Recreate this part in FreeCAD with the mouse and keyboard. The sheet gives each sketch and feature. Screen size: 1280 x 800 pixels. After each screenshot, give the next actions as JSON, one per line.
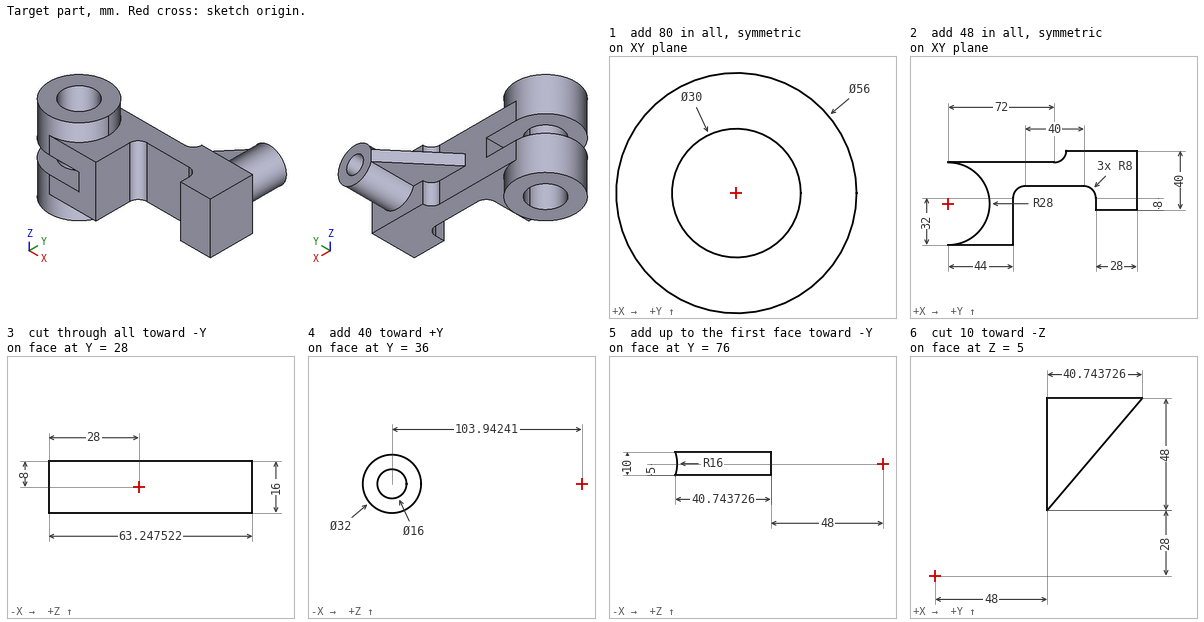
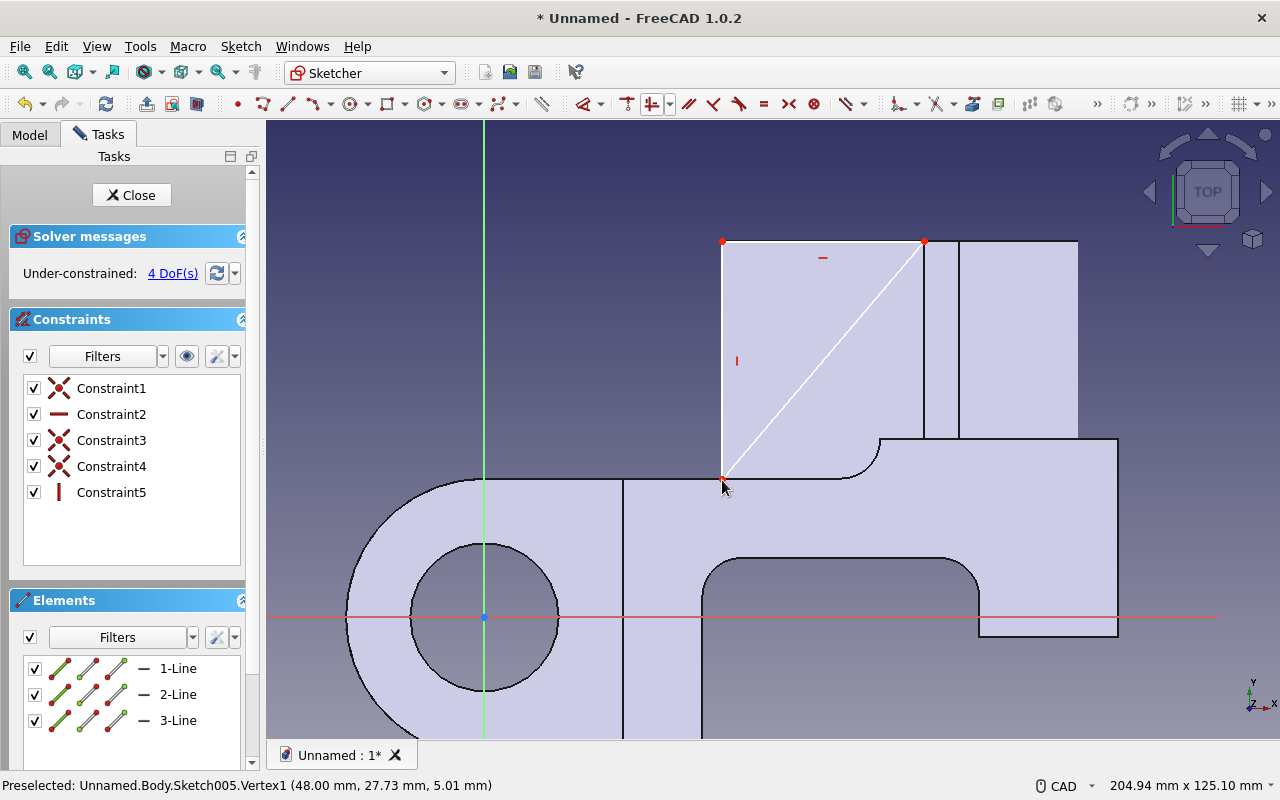
{"action": "left_click", "coordinate": [582, 104]}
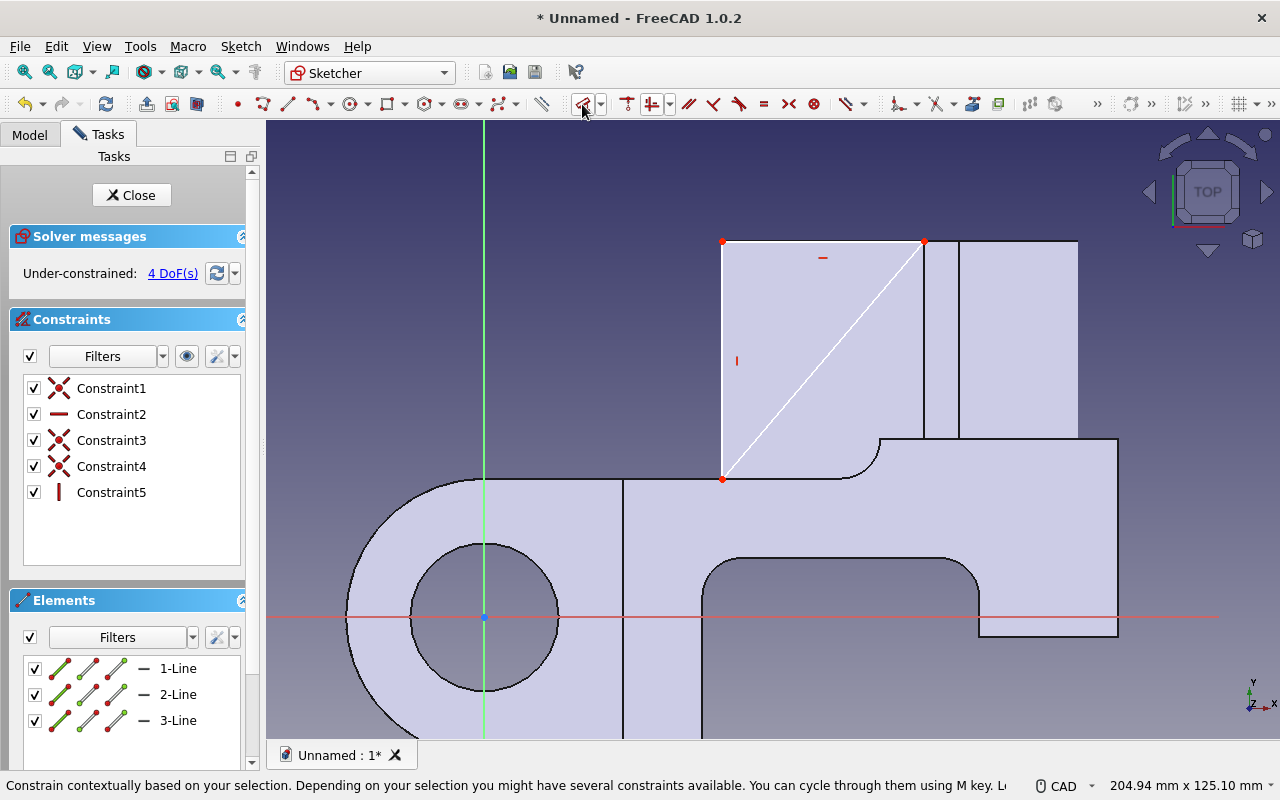
{"action": "left_click", "coordinate": [722, 313]}
{"action": "left_click", "coordinate": [756, 361]}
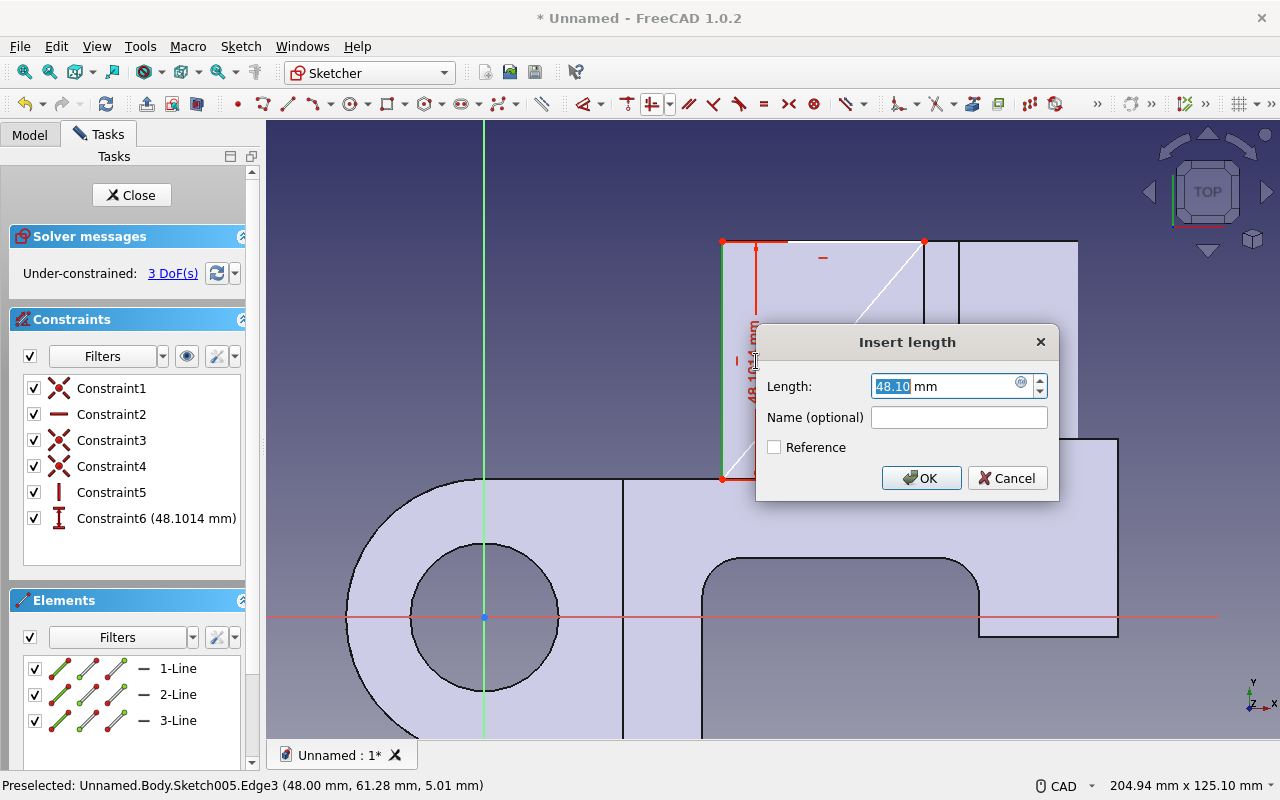
{"action": "type", "text": "48"}
{"action": "key", "text": "Return"}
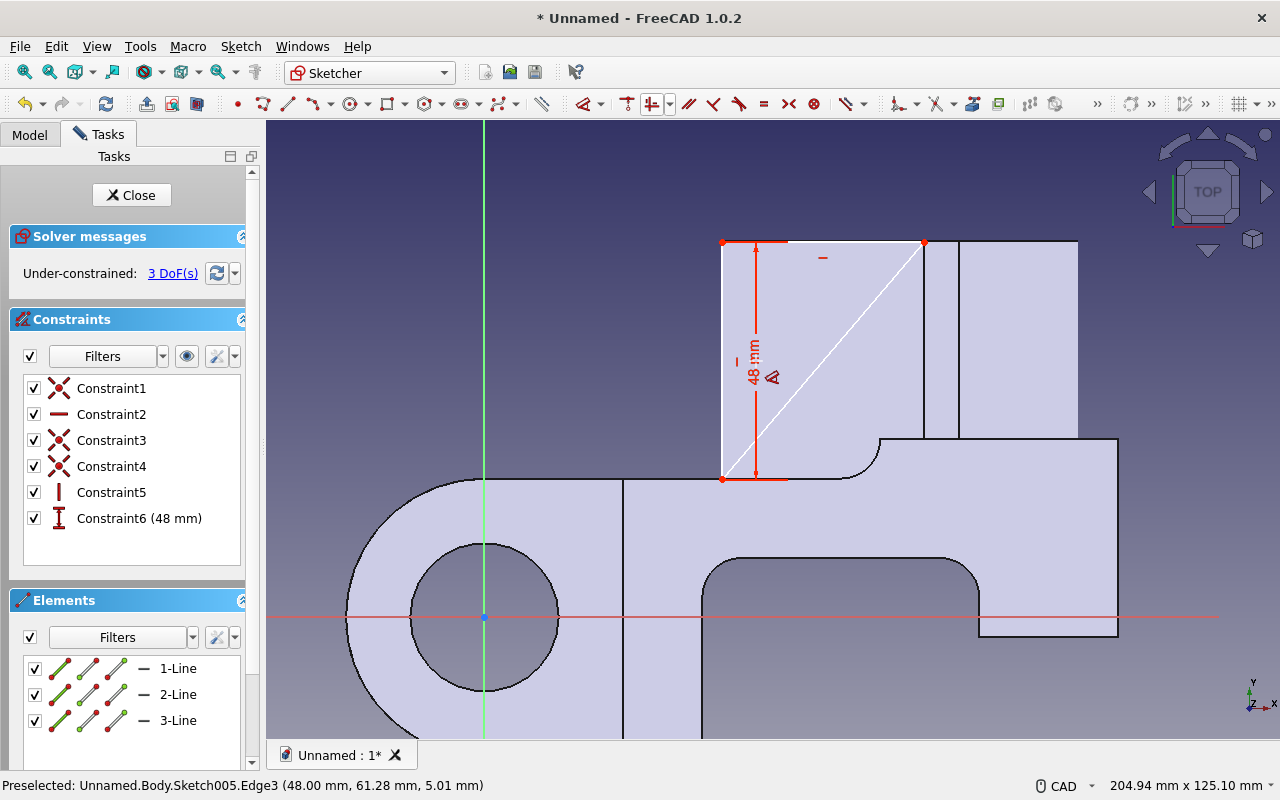
{"action": "left_click", "coordinate": [722, 480]}
{"action": "left_click", "coordinate": [603, 651]}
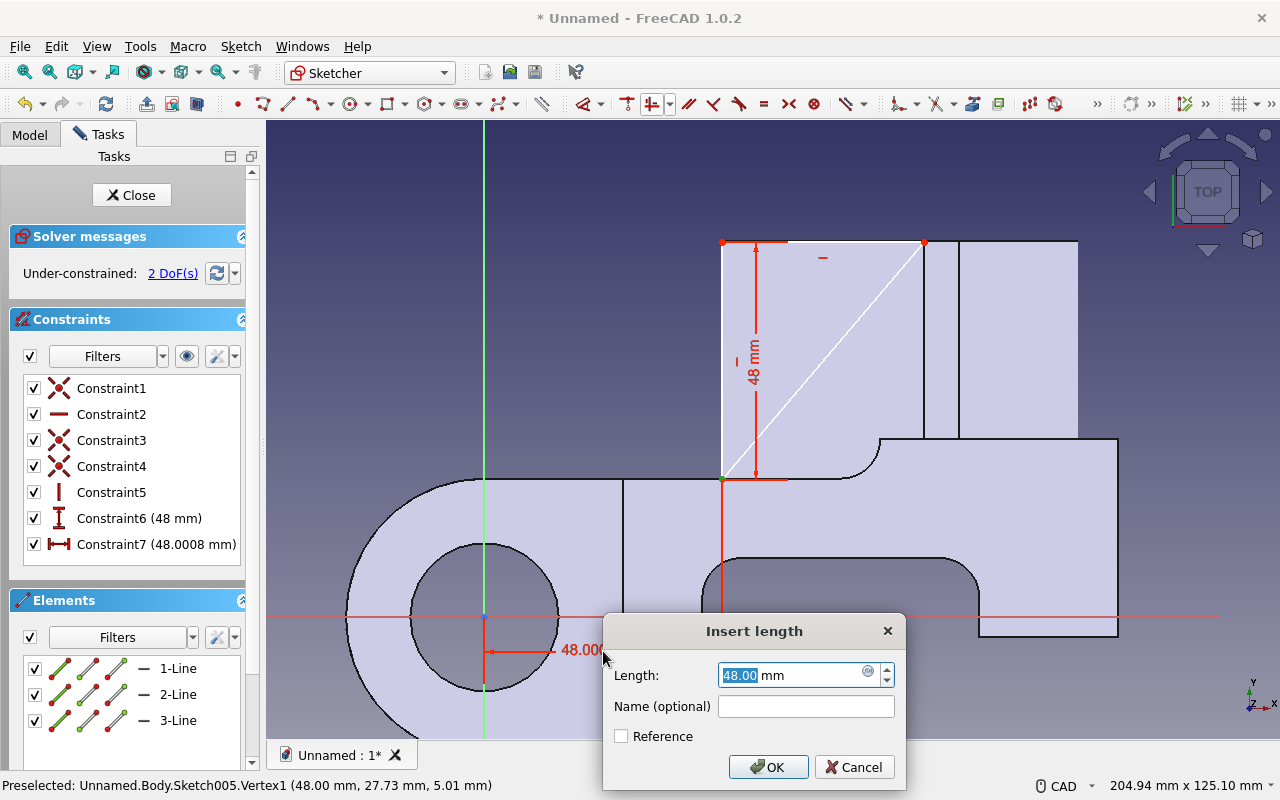
{"action": "type", "text": "48"}
{"action": "key", "text": "Return"}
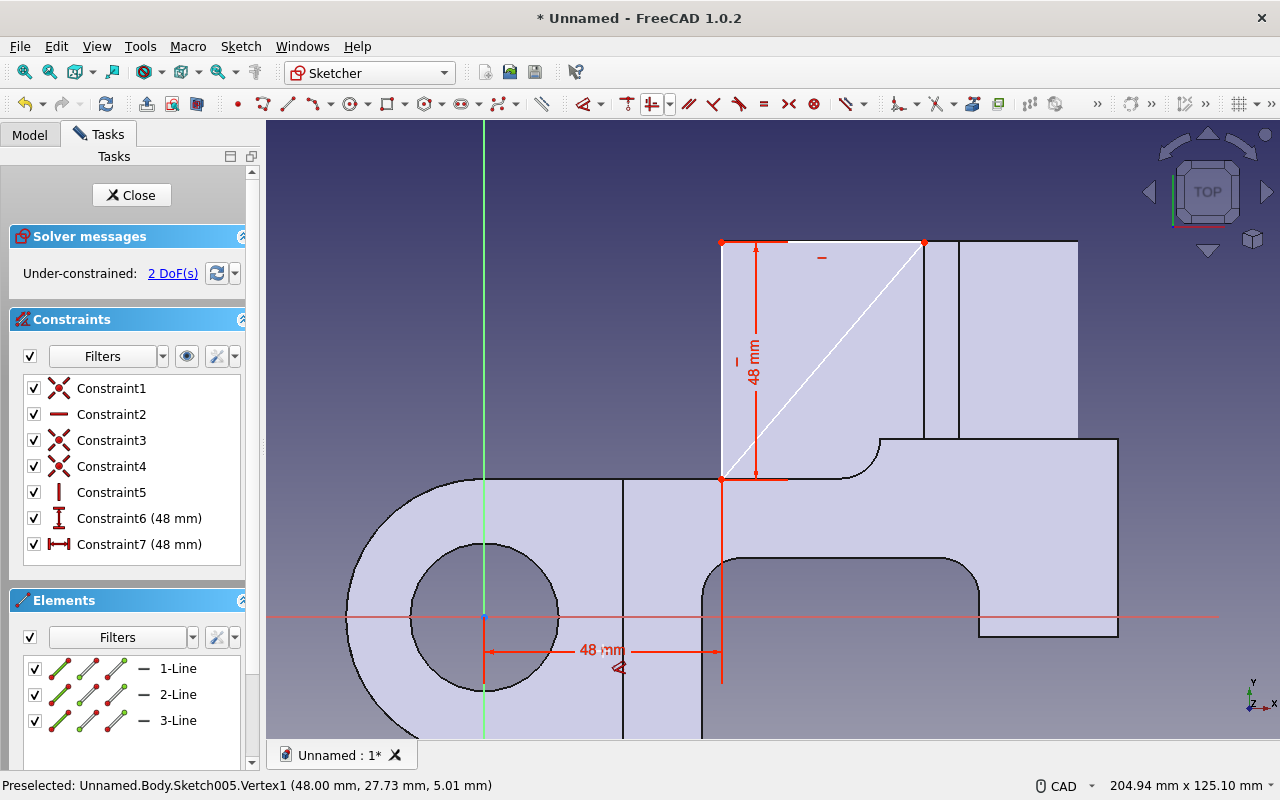
{"action": "left_click", "coordinate": [722, 480]}
{"action": "left_click", "coordinate": [450, 549]}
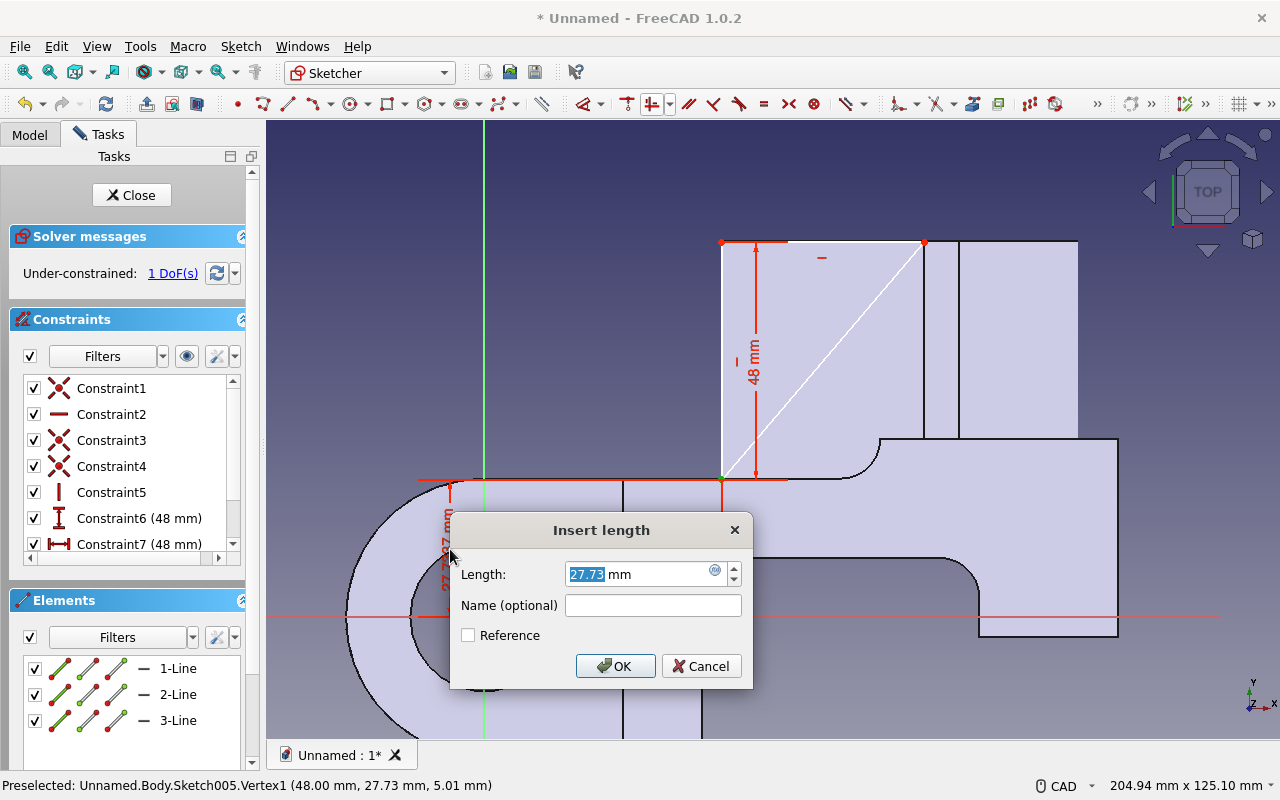
{"action": "type", "text": "28"}
{"action": "key", "text": "Return"}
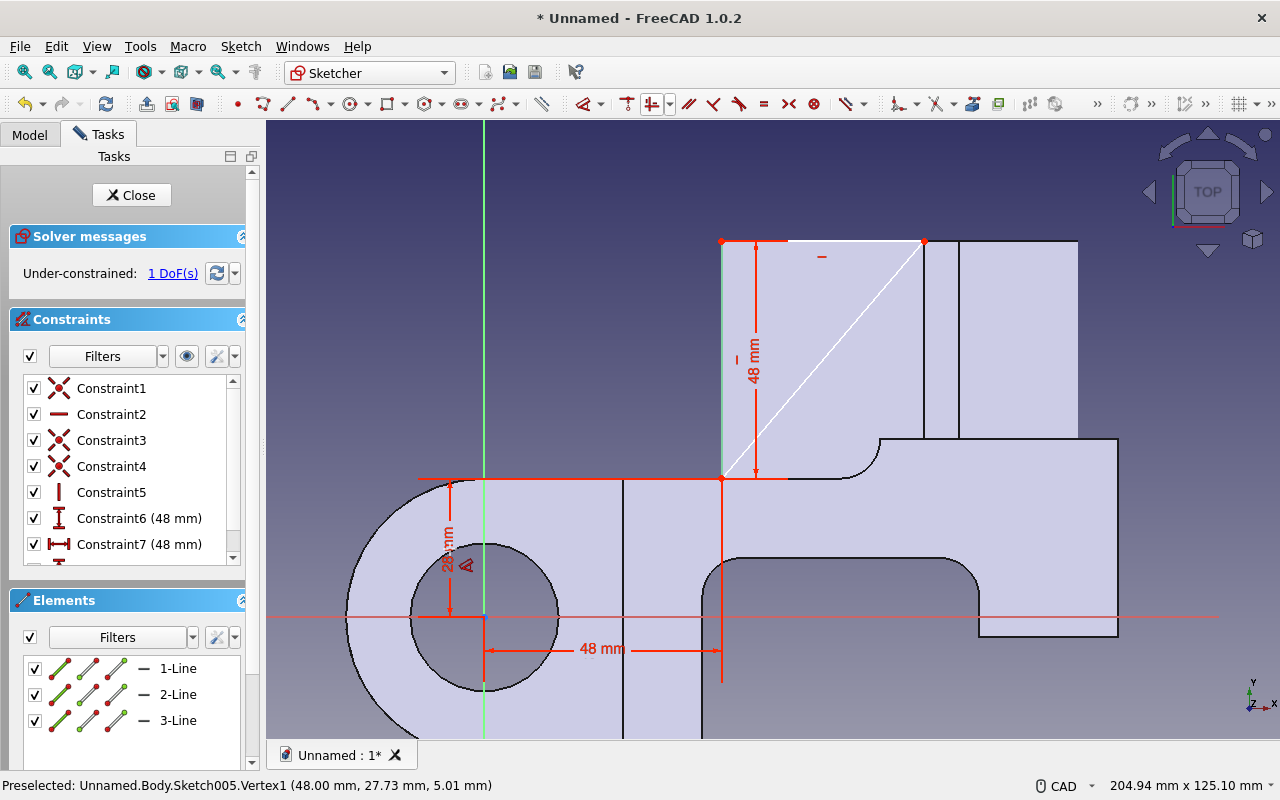
{"action": "left_click", "coordinate": [863, 241]}
{"action": "left_click", "coordinate": [823, 207]}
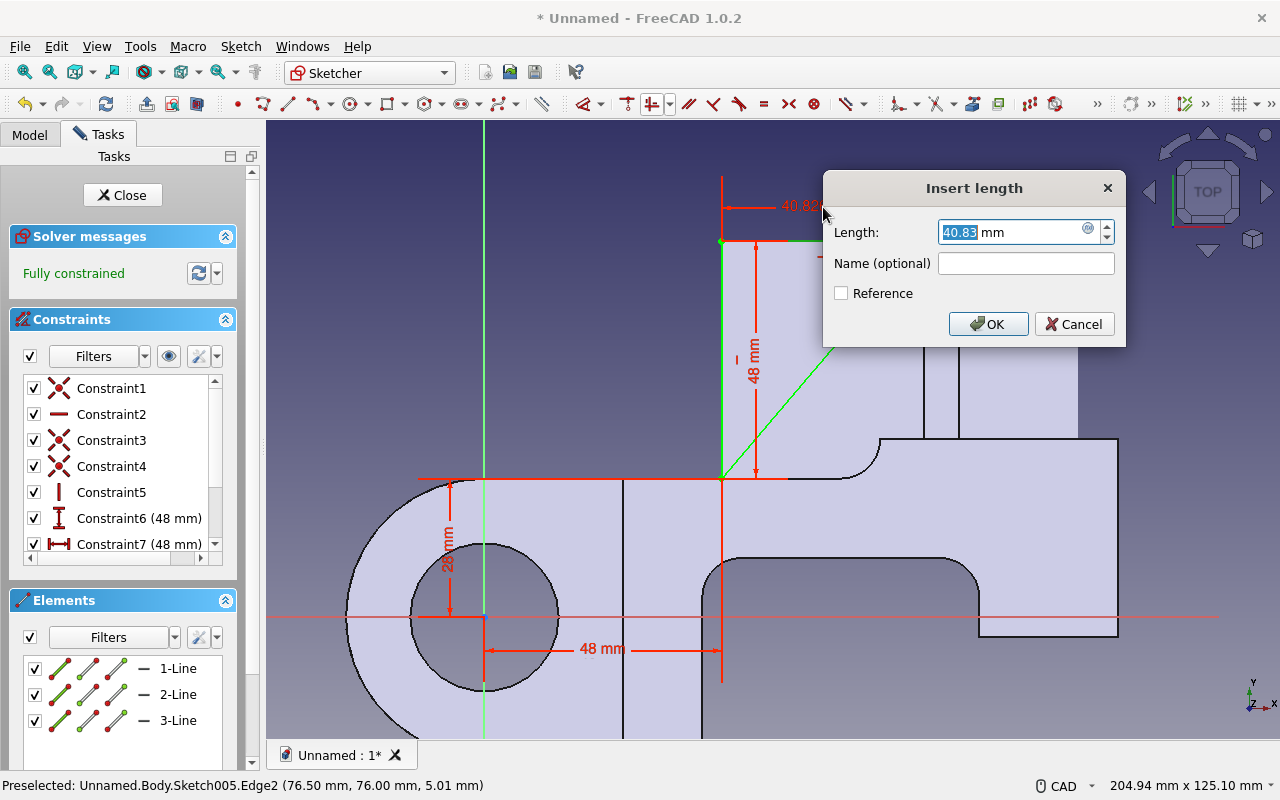
{"action": "type", "text": "40.743726"}
{"action": "key", "text": "Return"}
{"action": "key", "text": "Escape"}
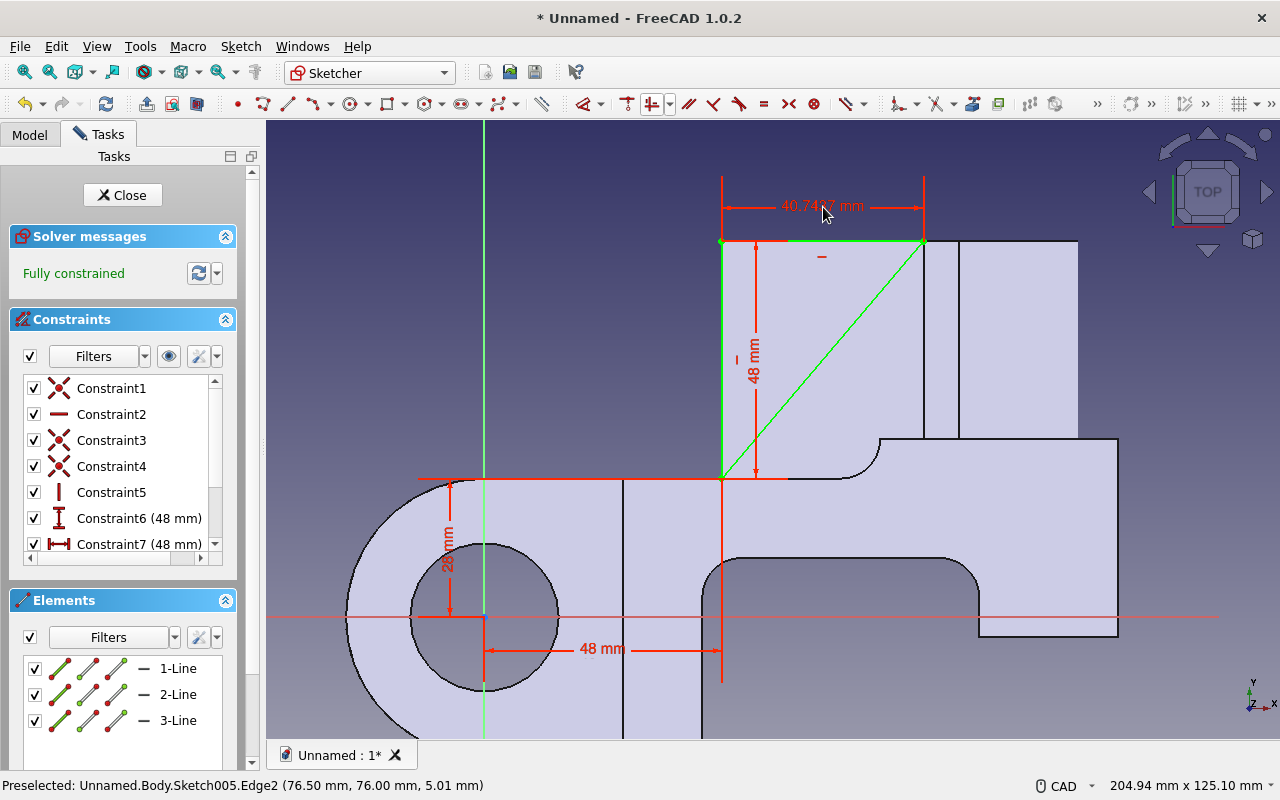
{"action": "left_click", "coordinate": [123, 195]}